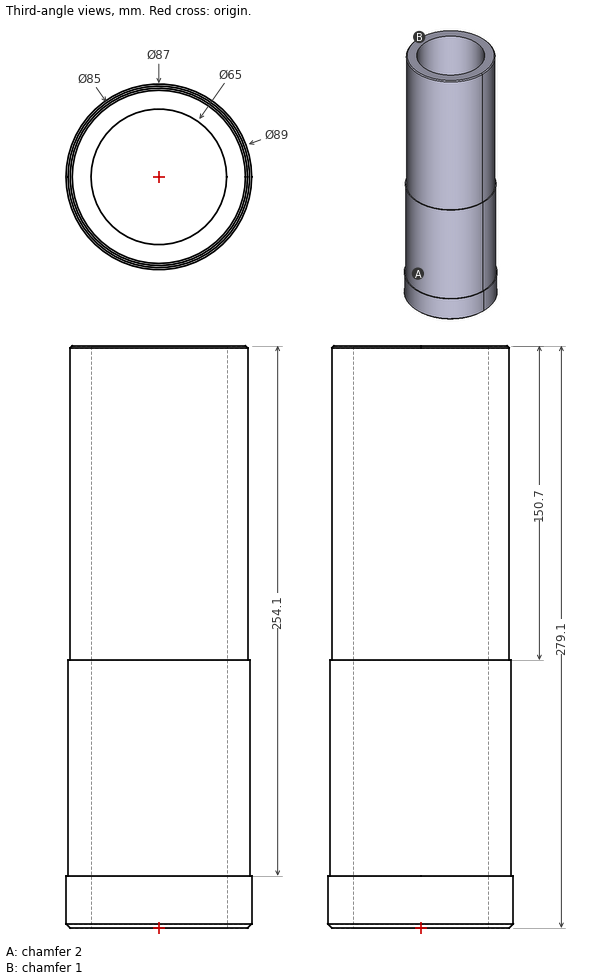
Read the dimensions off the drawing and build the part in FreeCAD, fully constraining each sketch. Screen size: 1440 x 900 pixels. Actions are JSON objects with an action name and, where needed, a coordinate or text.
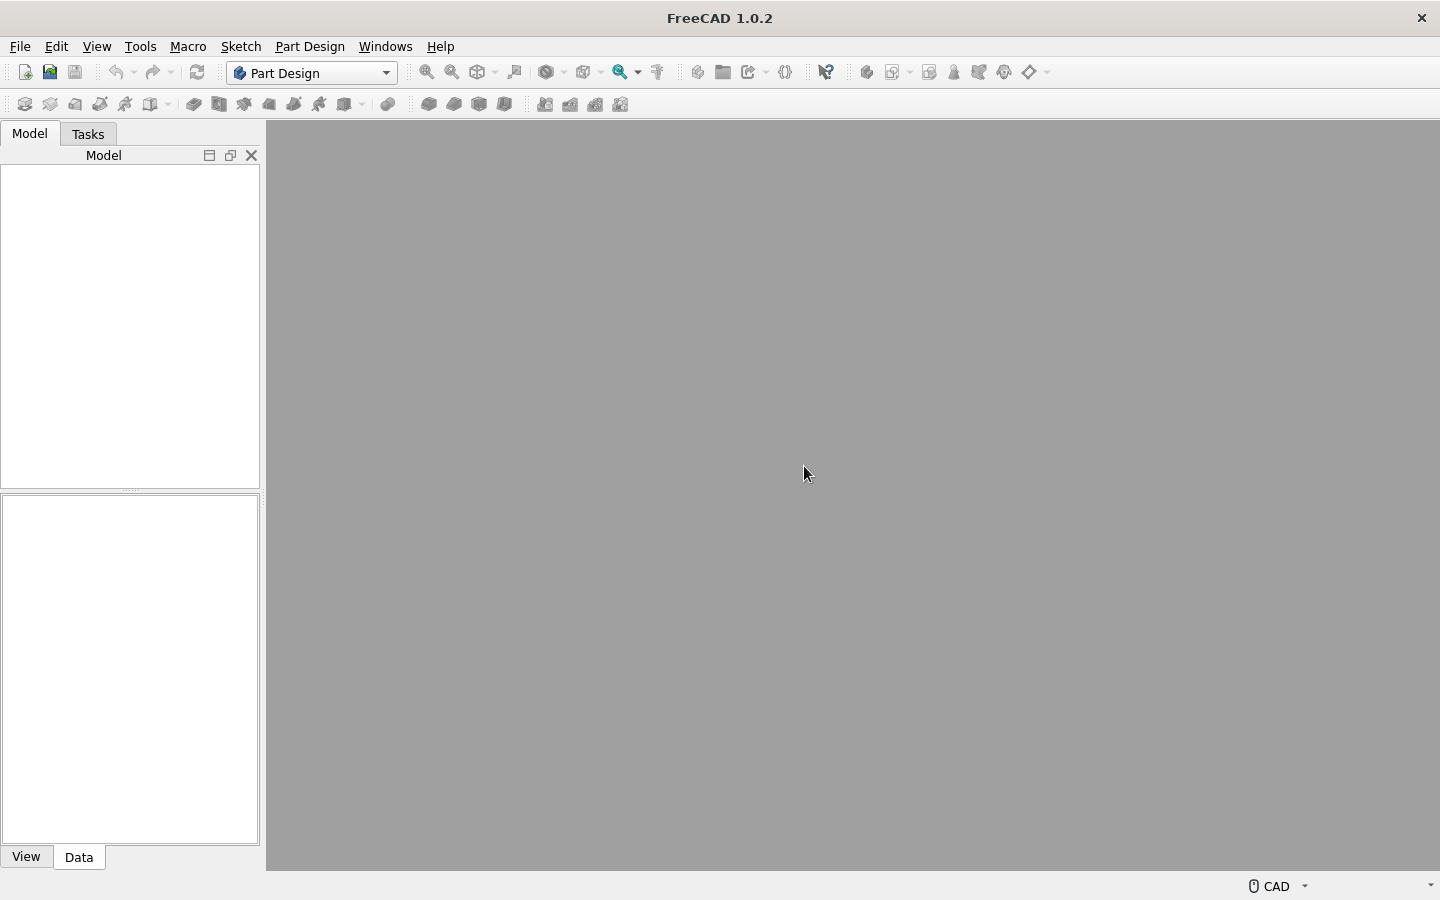
{"action": "left_click", "coordinate": [25, 72]}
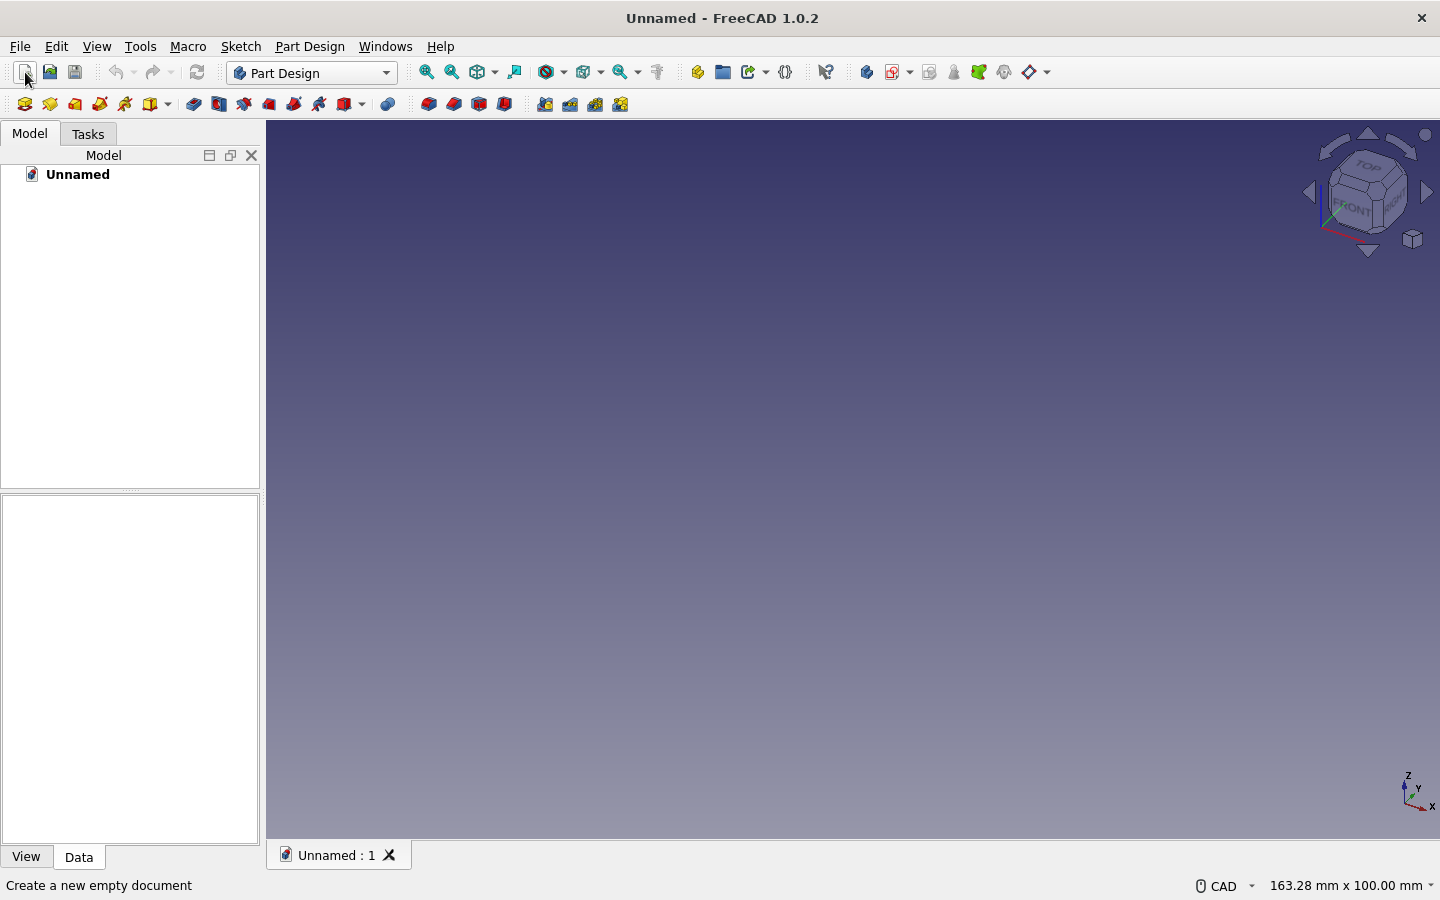
{"action": "left_click", "coordinate": [892, 72]}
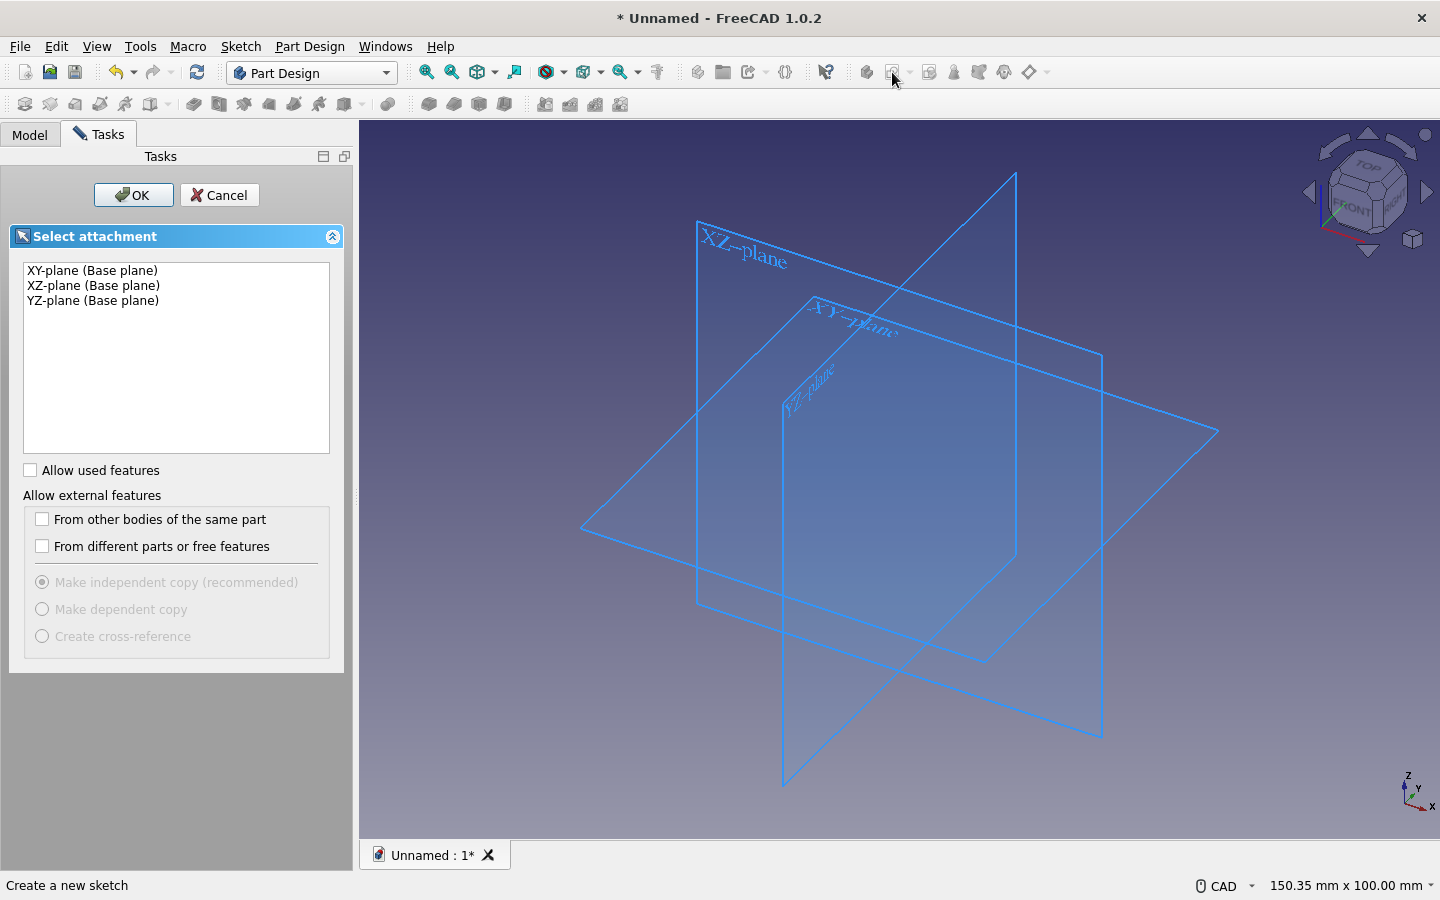
{"action": "left_click", "coordinate": [84, 270]}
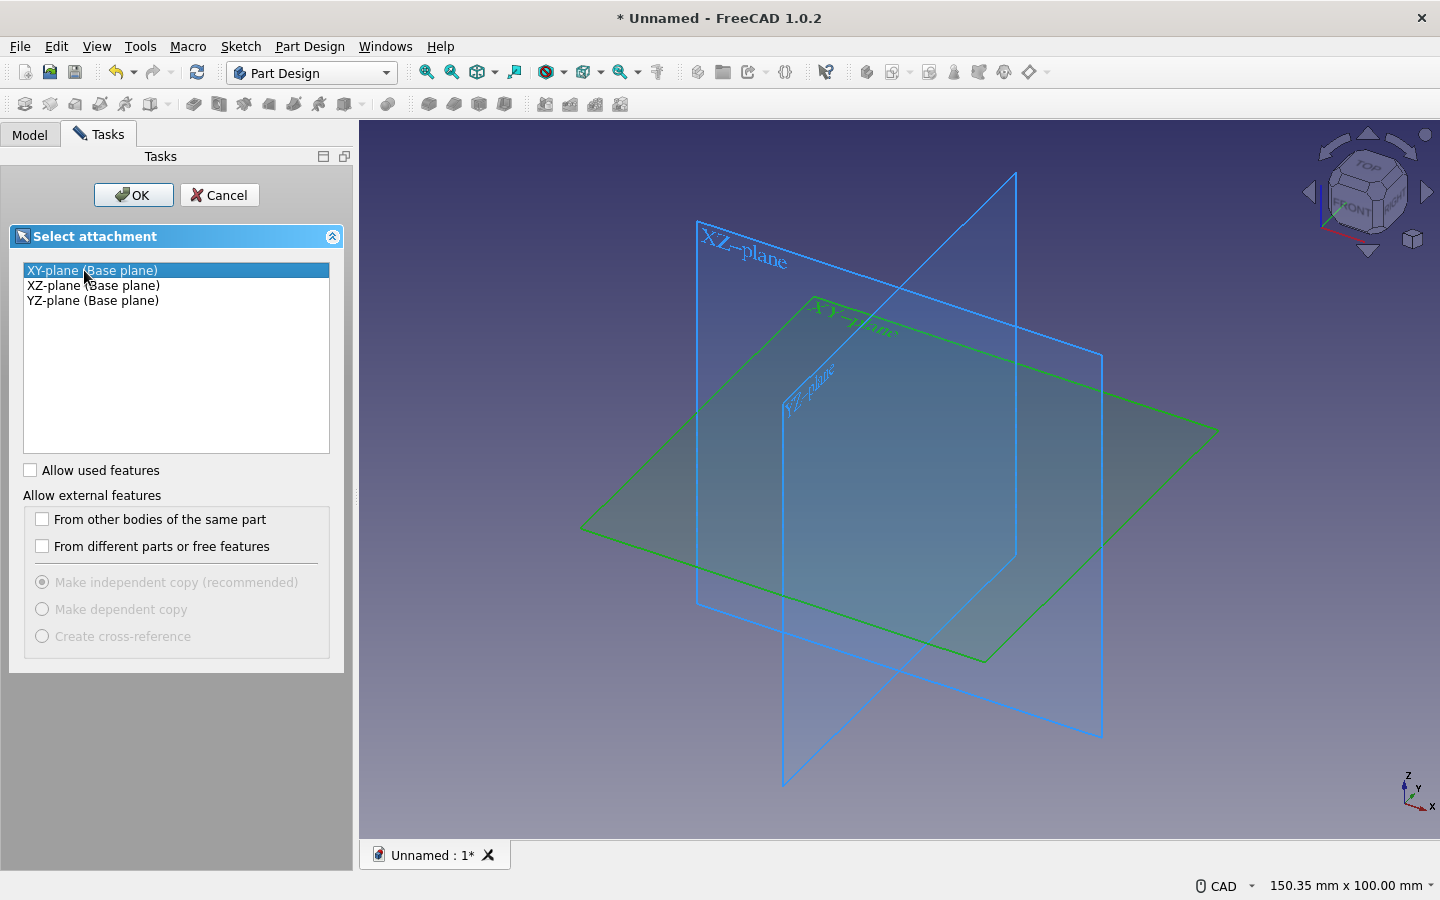
{"action": "left_click", "coordinate": [134, 195]}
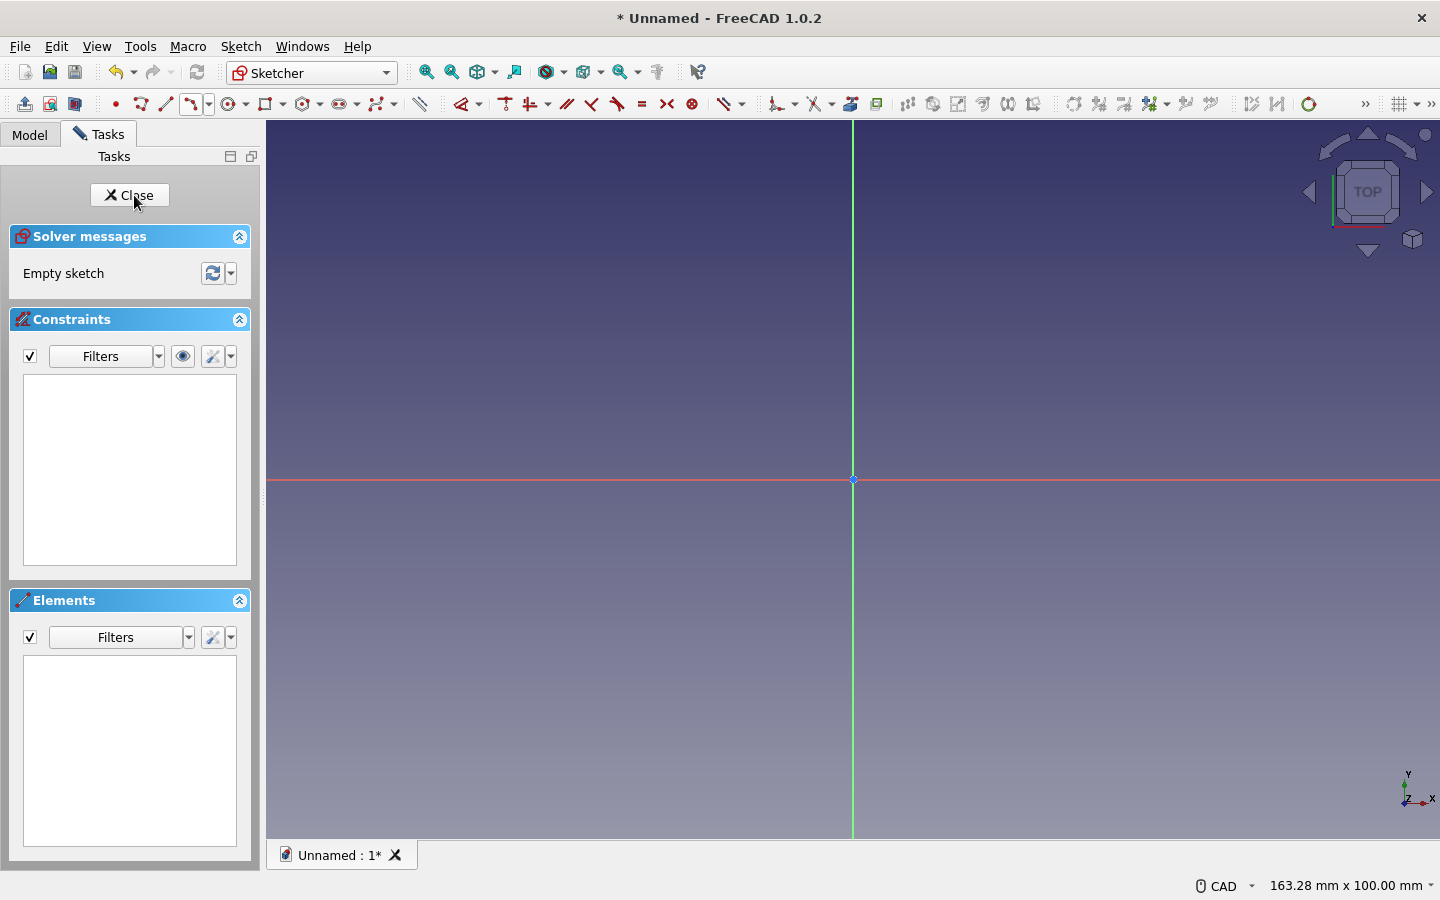
{"action": "scroll", "coordinate": [645, 480], "scroll_direction": "down", "scroll_amount": 2}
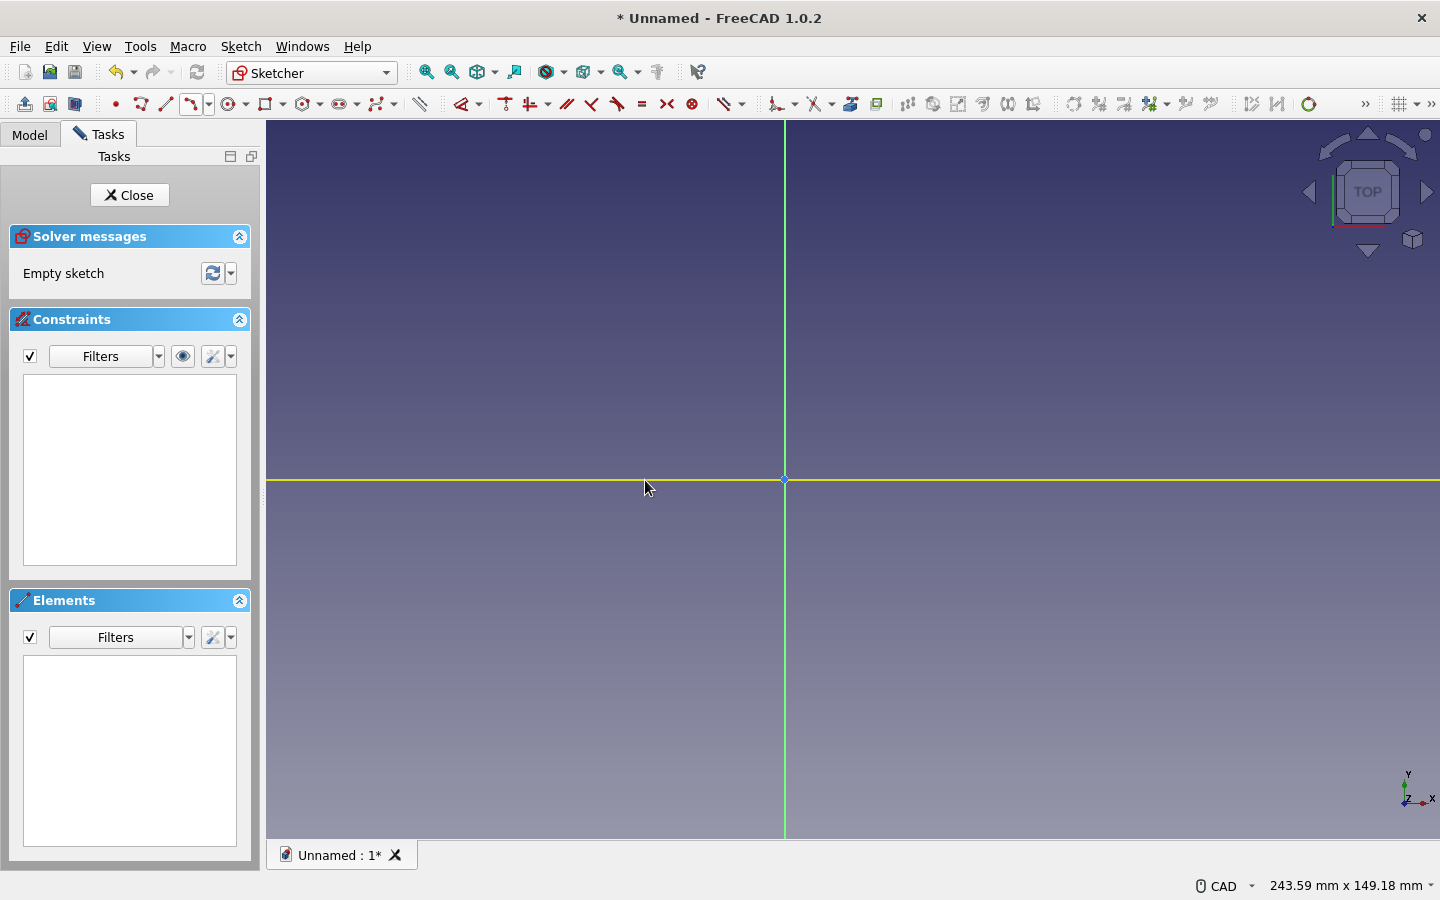
{"action": "left_click", "coordinate": [228, 104]}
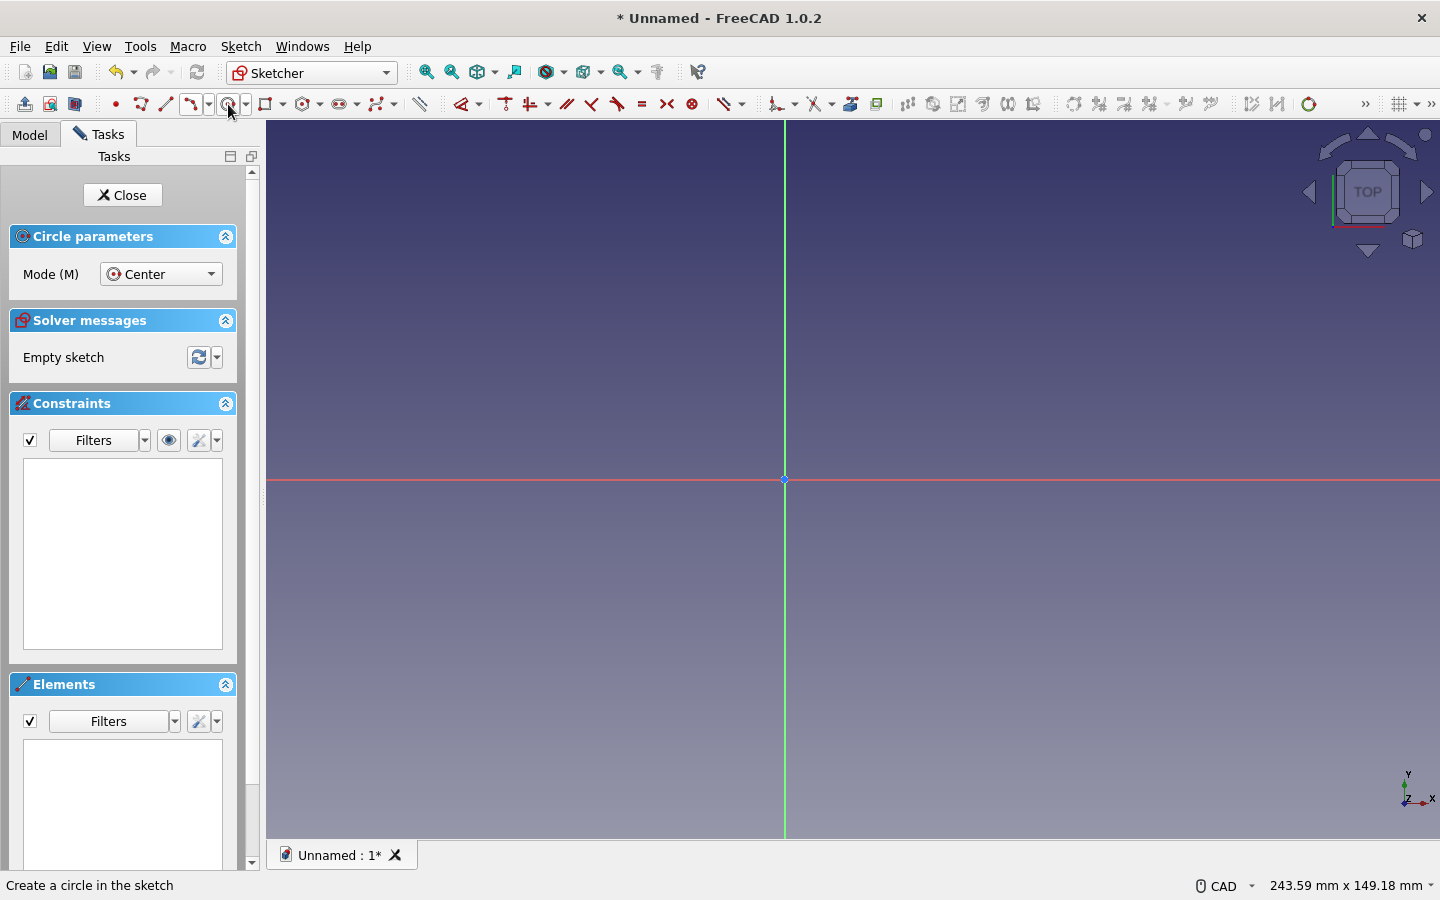
{"action": "left_click", "coordinate": [785, 480]}
{"action": "mouse_move", "coordinate": [936, 328]}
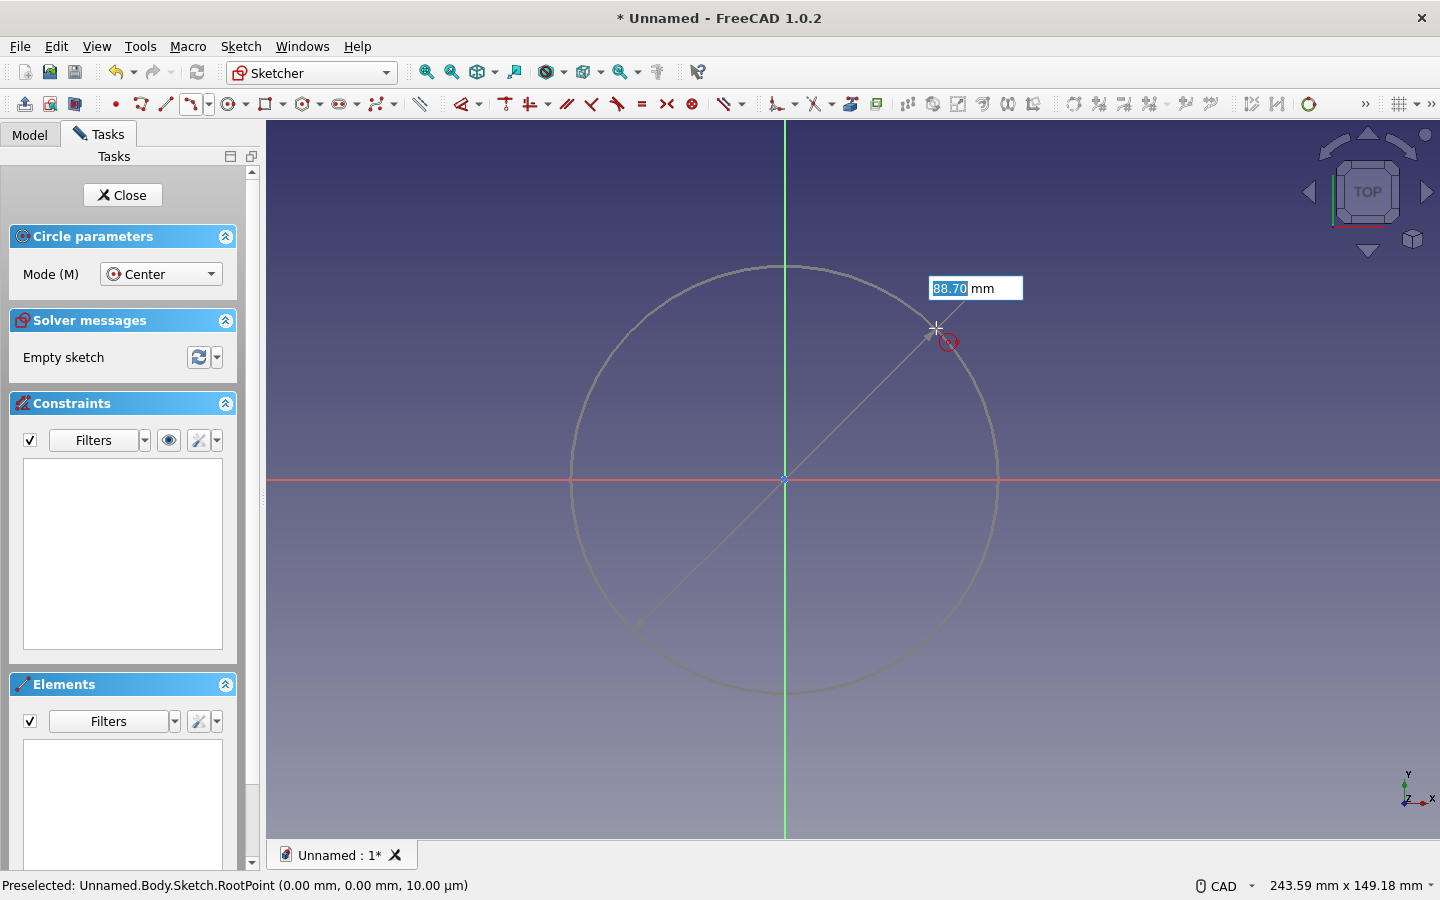
{"action": "type", "text": "89"}
{"action": "key", "text": "Return"}